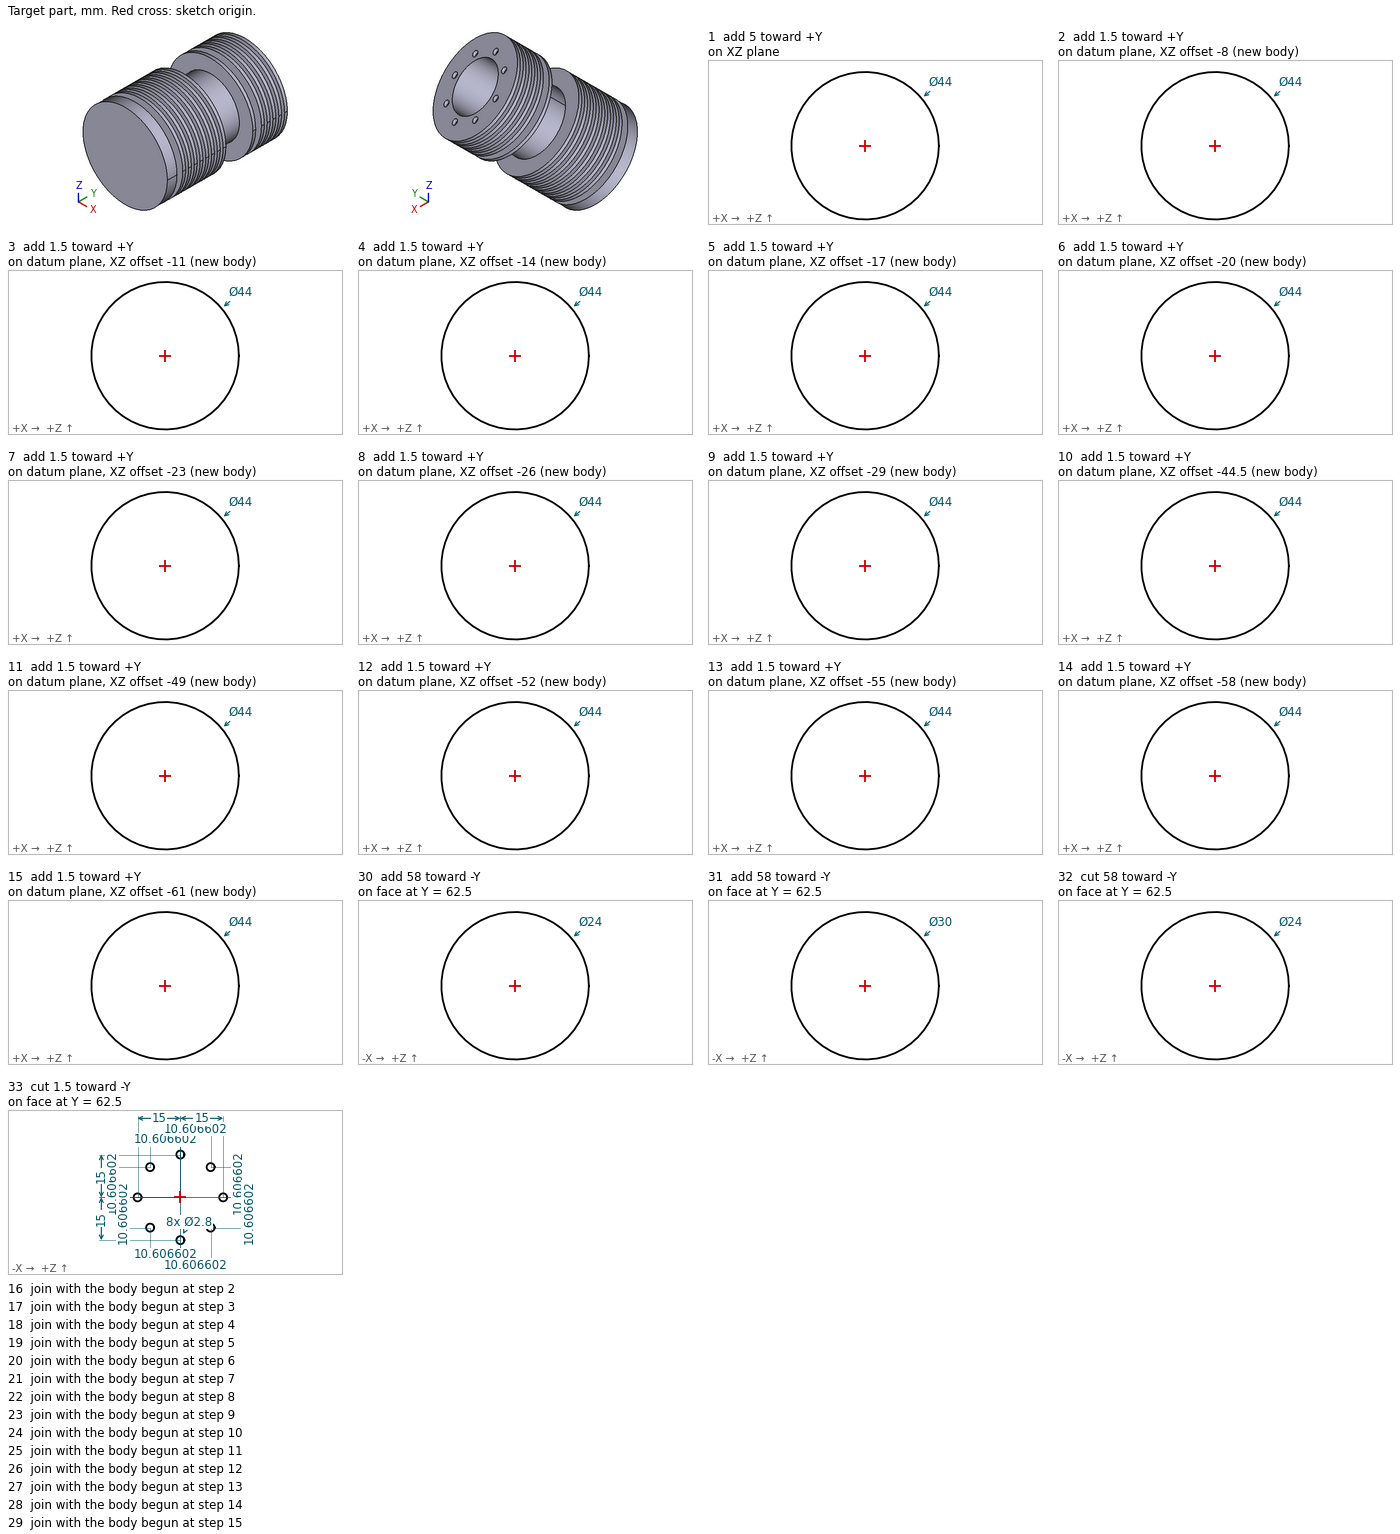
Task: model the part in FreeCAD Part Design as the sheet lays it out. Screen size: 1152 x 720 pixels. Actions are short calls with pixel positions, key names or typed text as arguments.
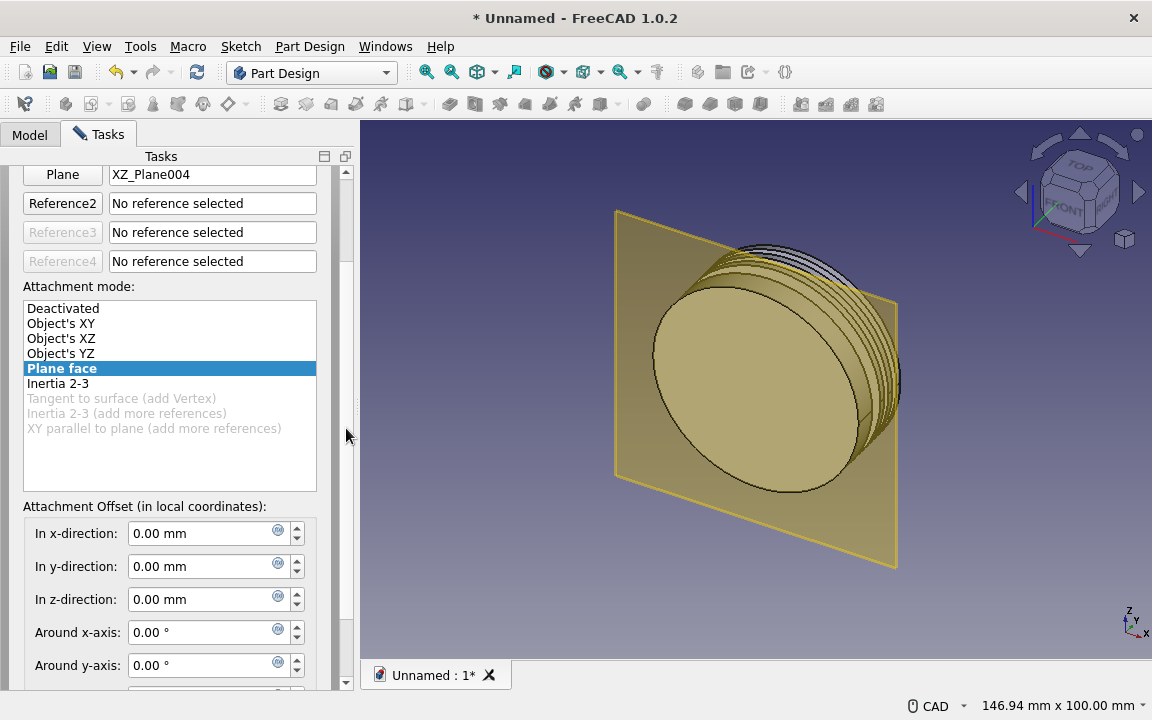
triple_click(210, 600)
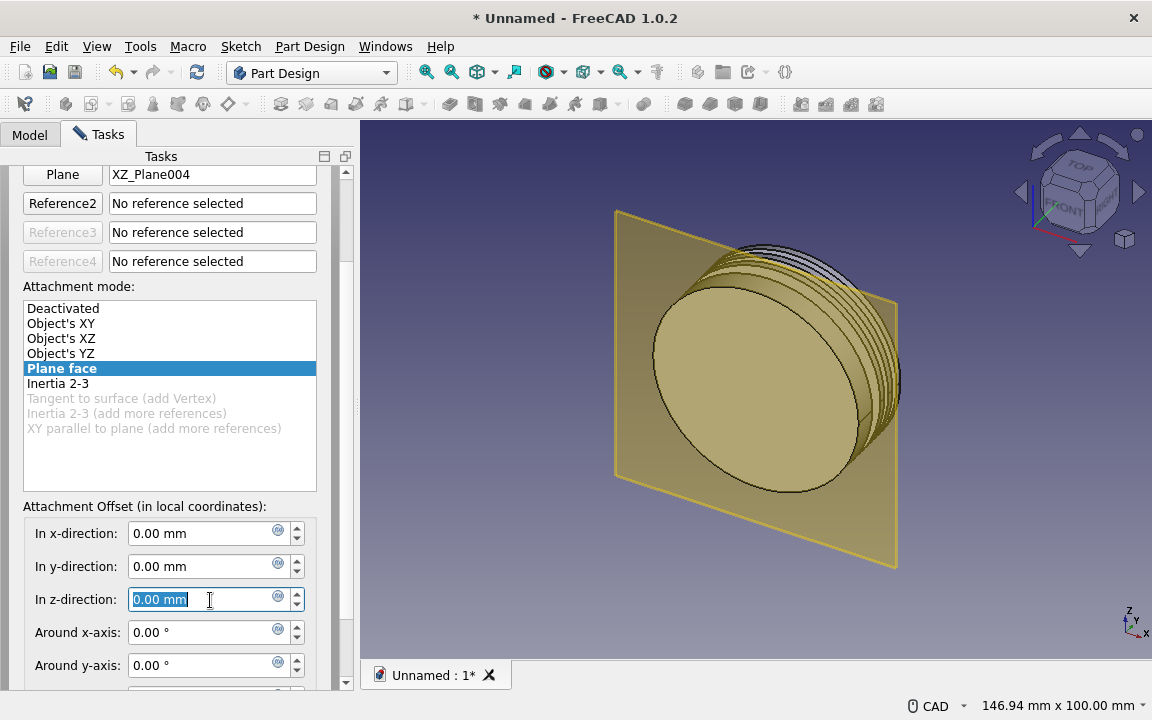
text(-17)
key(Tab)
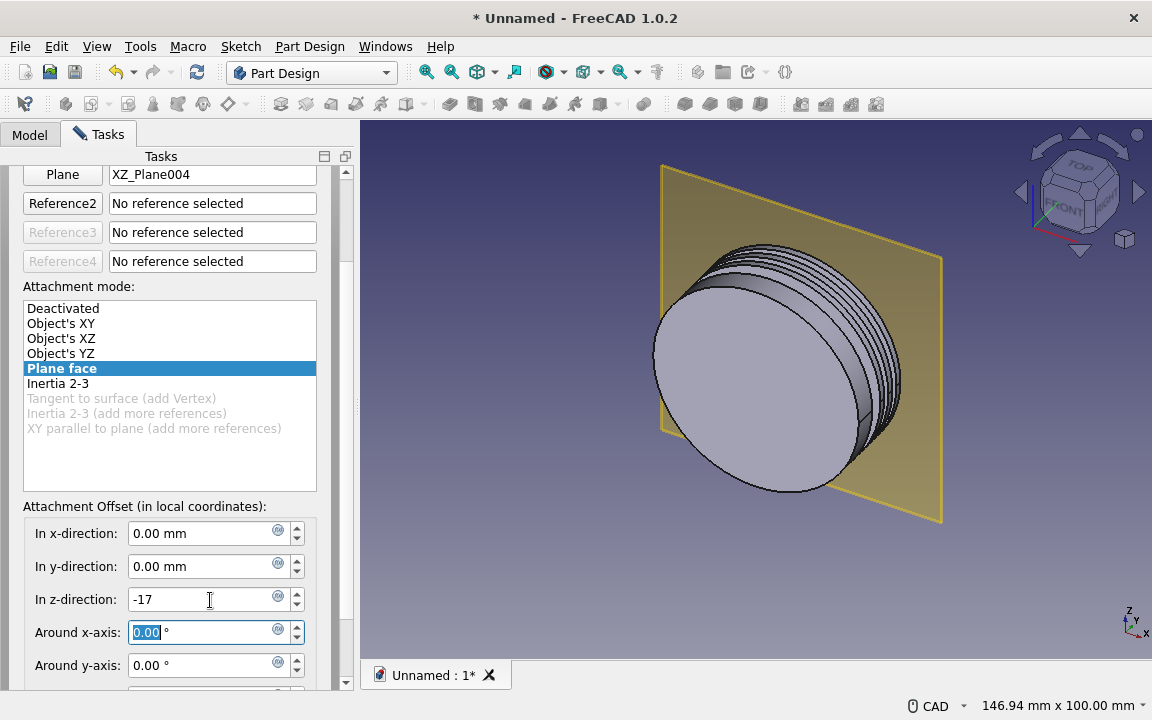
scroll(346, 428, up, 3)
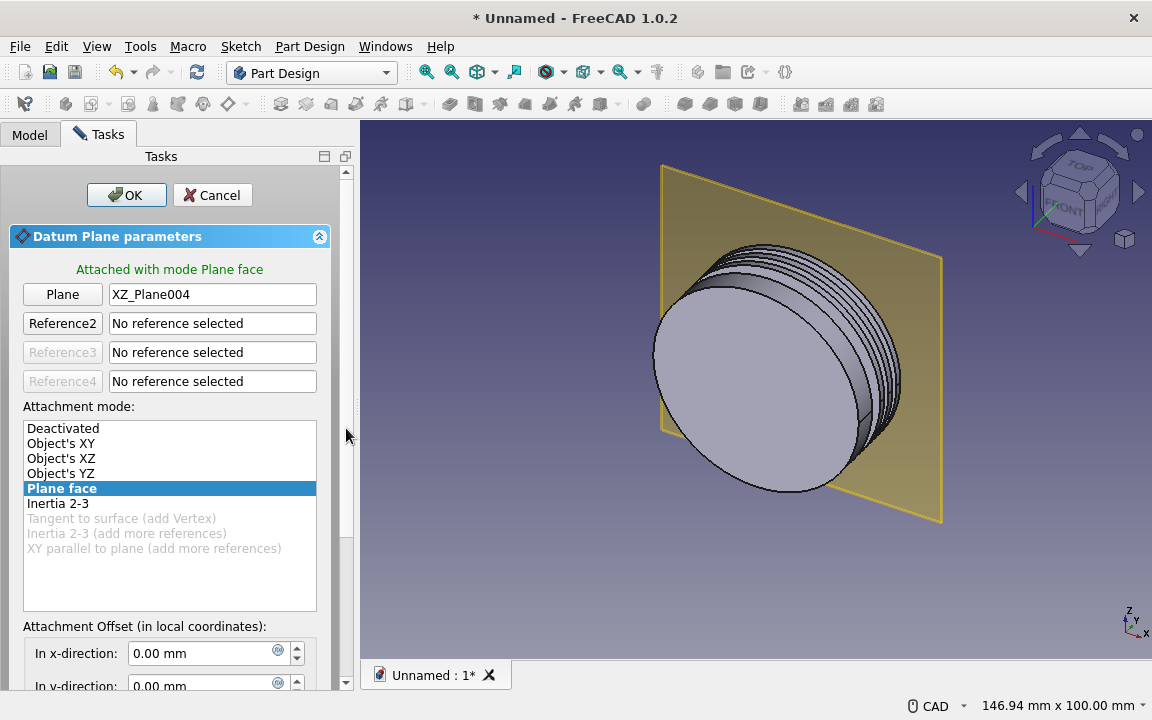
click(127, 195)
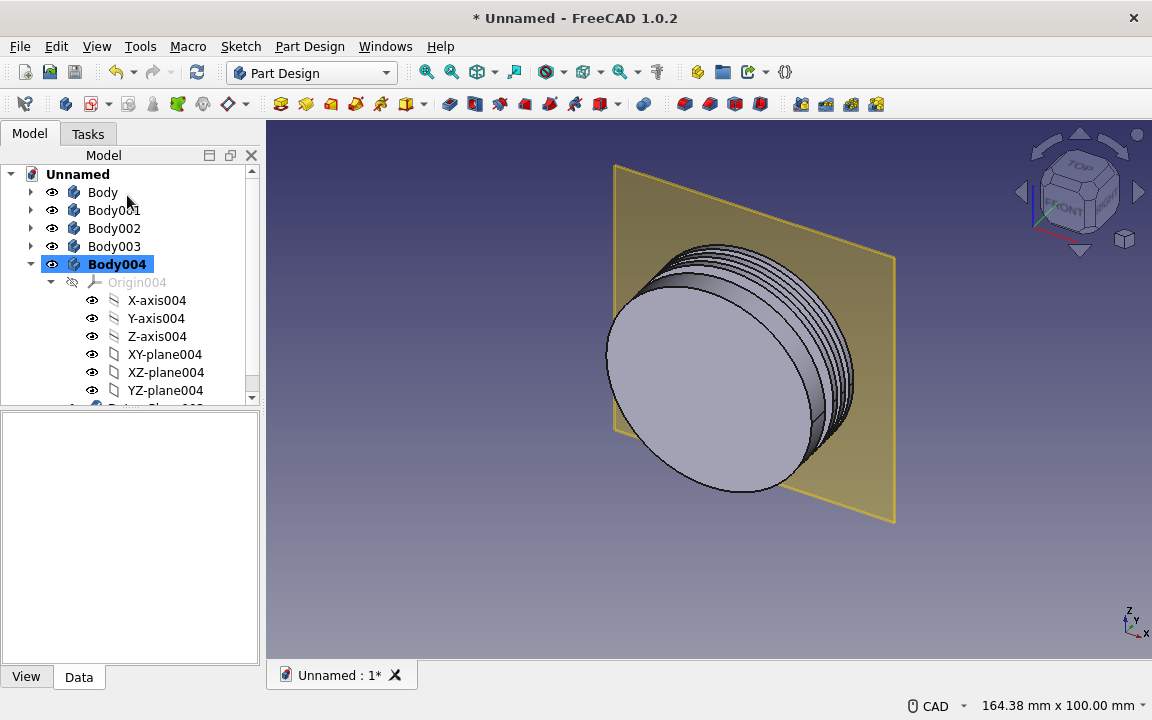
scroll(101, 278, down, 3)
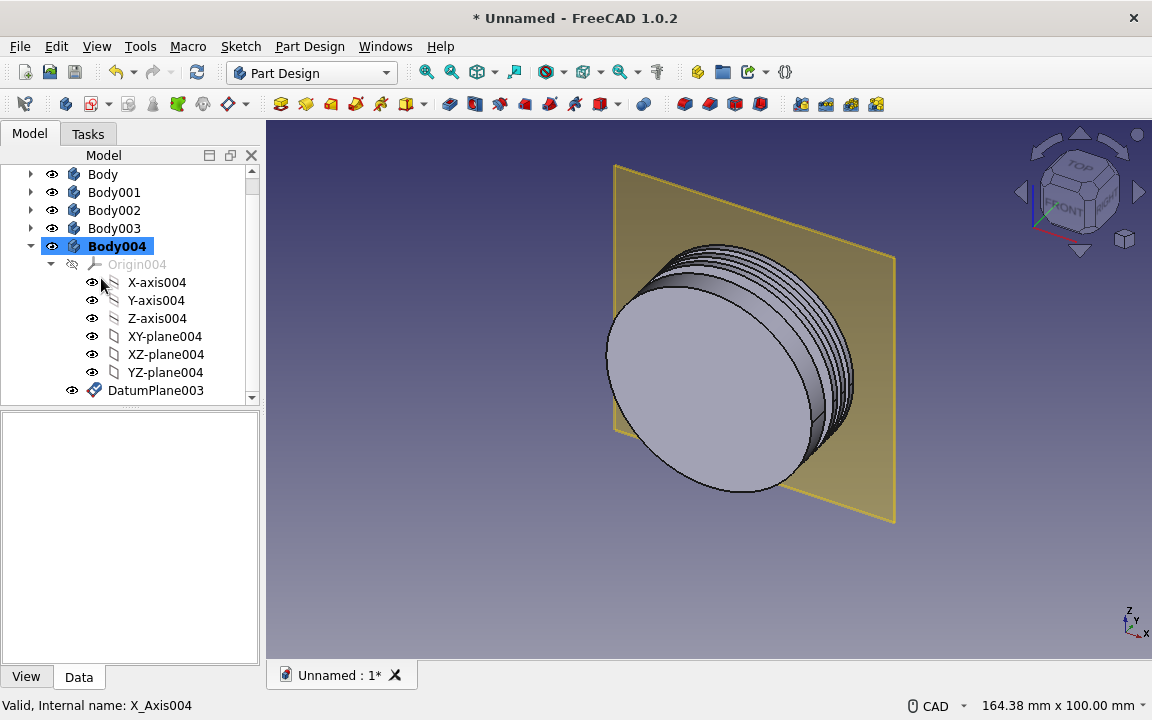
click(117, 390)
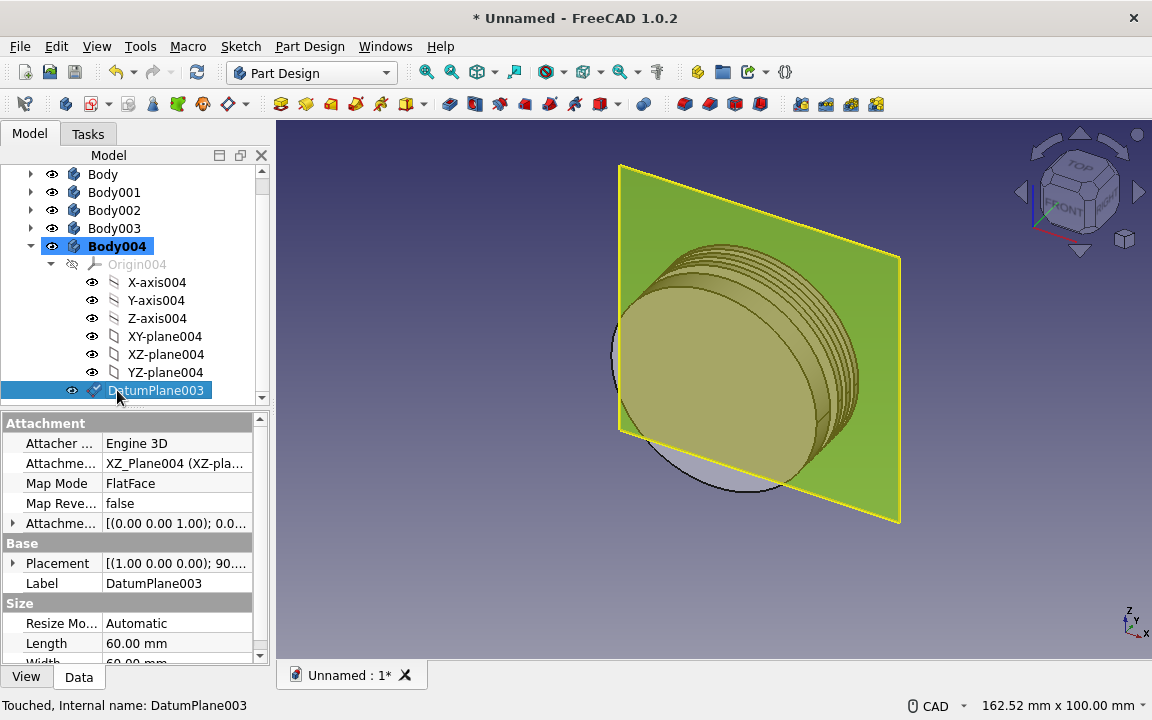
click(90, 104)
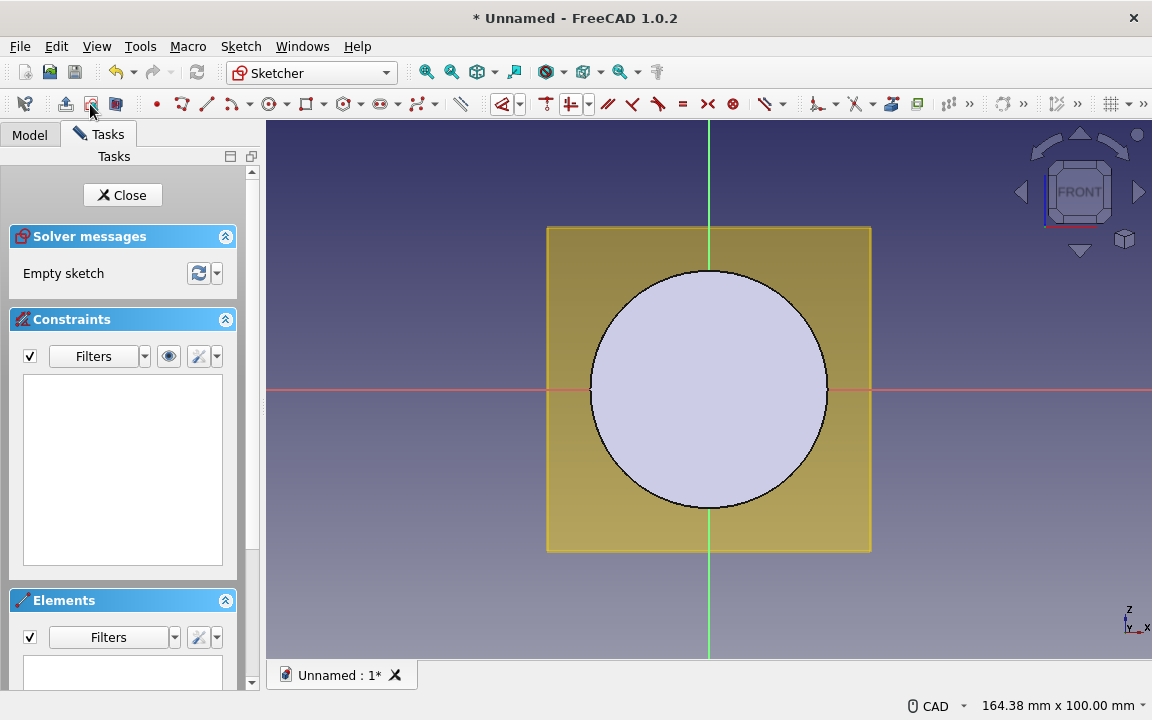
scroll(848, 390, up, 2)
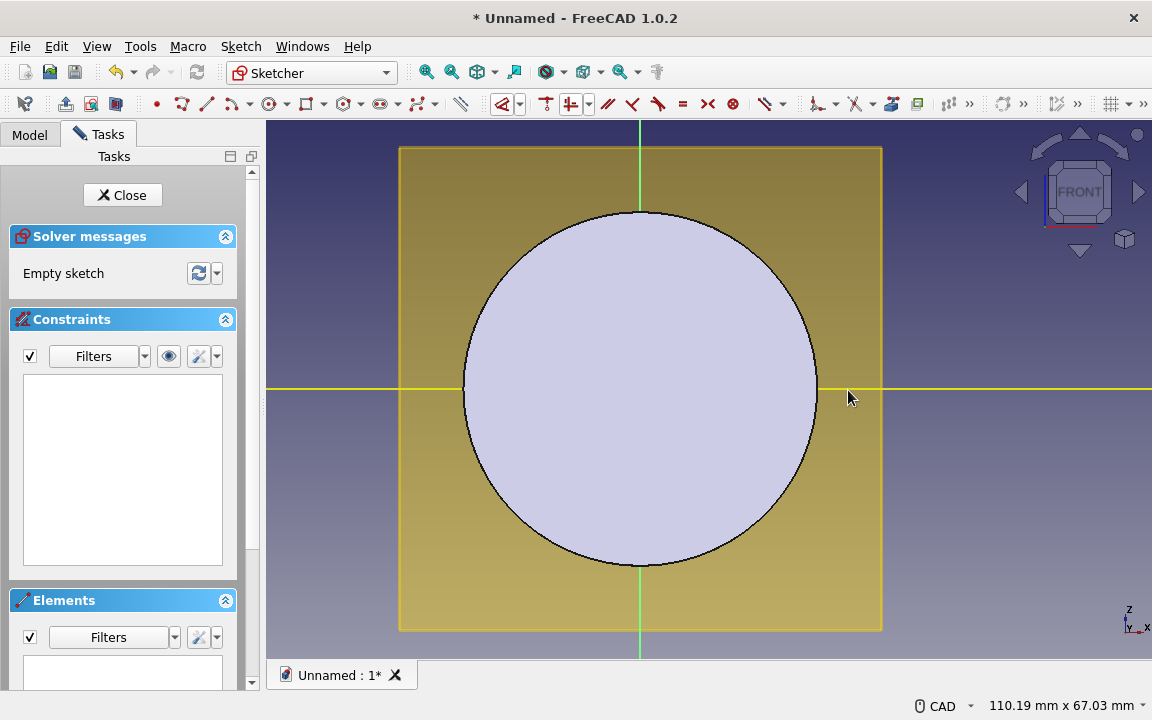
key(g)
key(c)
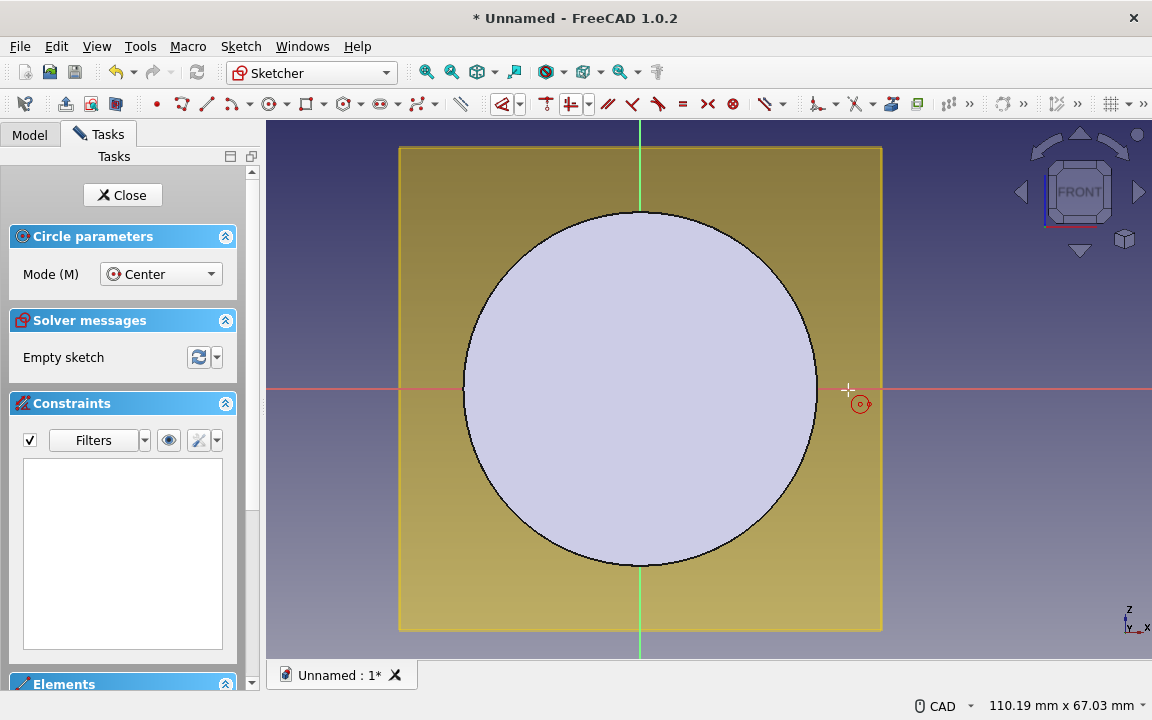
click(640, 389)
click(765, 264)
key(Escape)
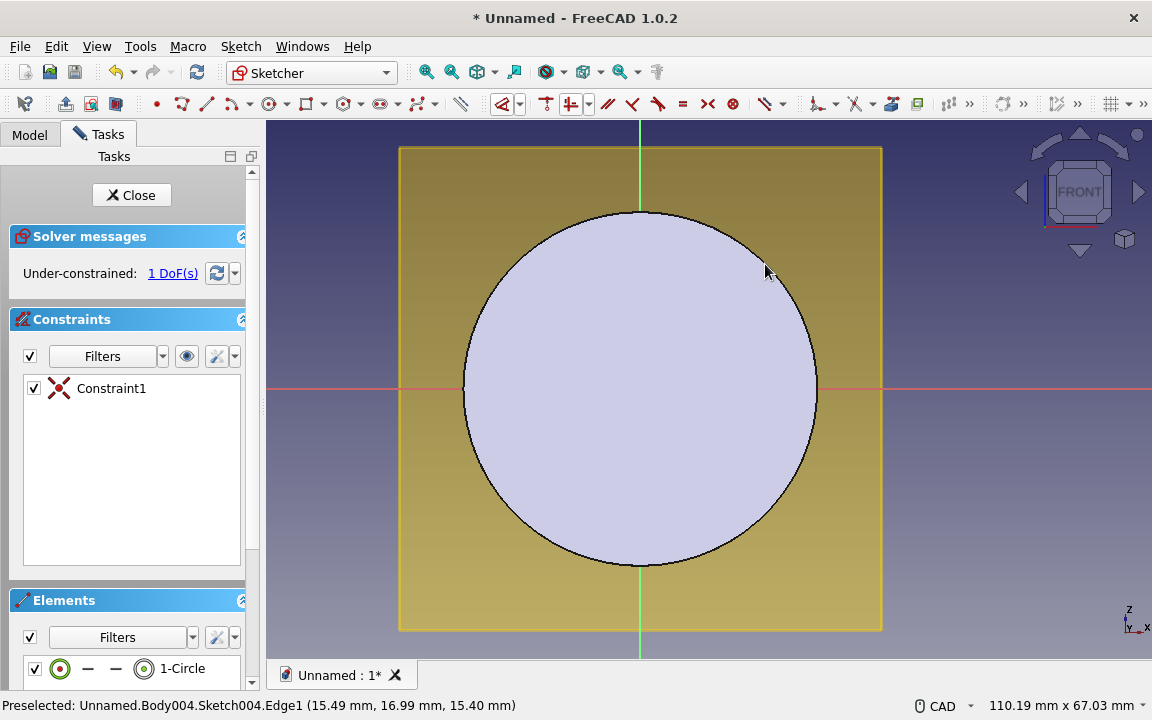
click(764, 264)